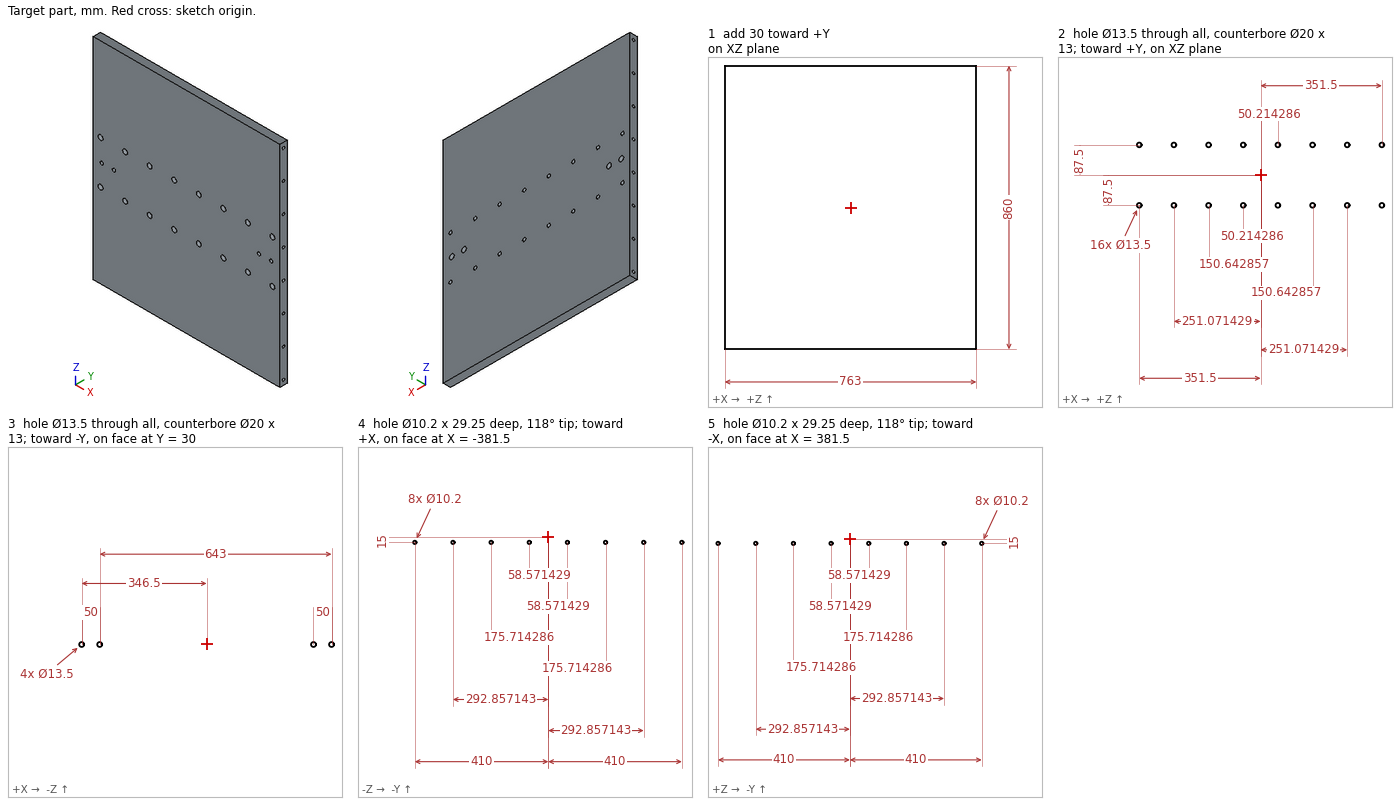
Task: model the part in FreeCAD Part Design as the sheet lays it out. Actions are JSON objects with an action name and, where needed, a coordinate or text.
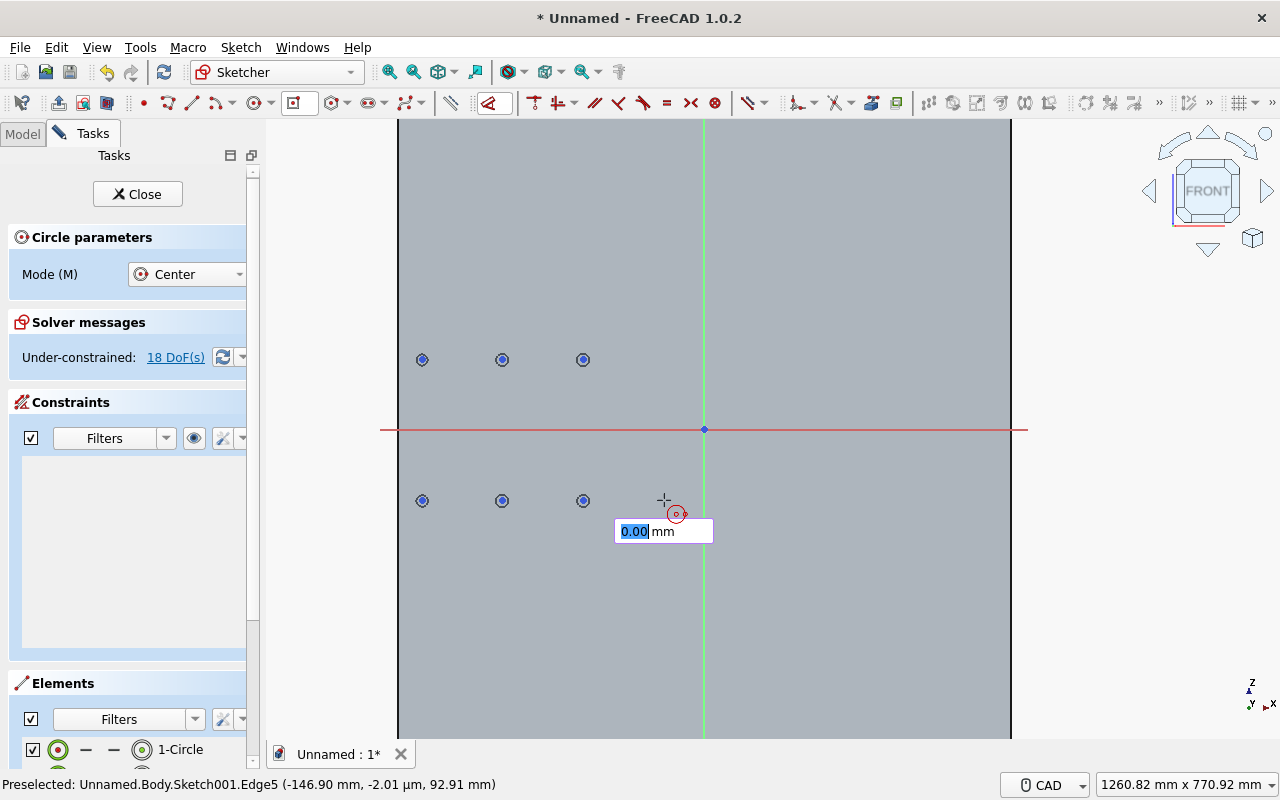
{"action": "scroll", "coordinate": [668, 496], "scroll_direction": "up", "scroll_amount": 6}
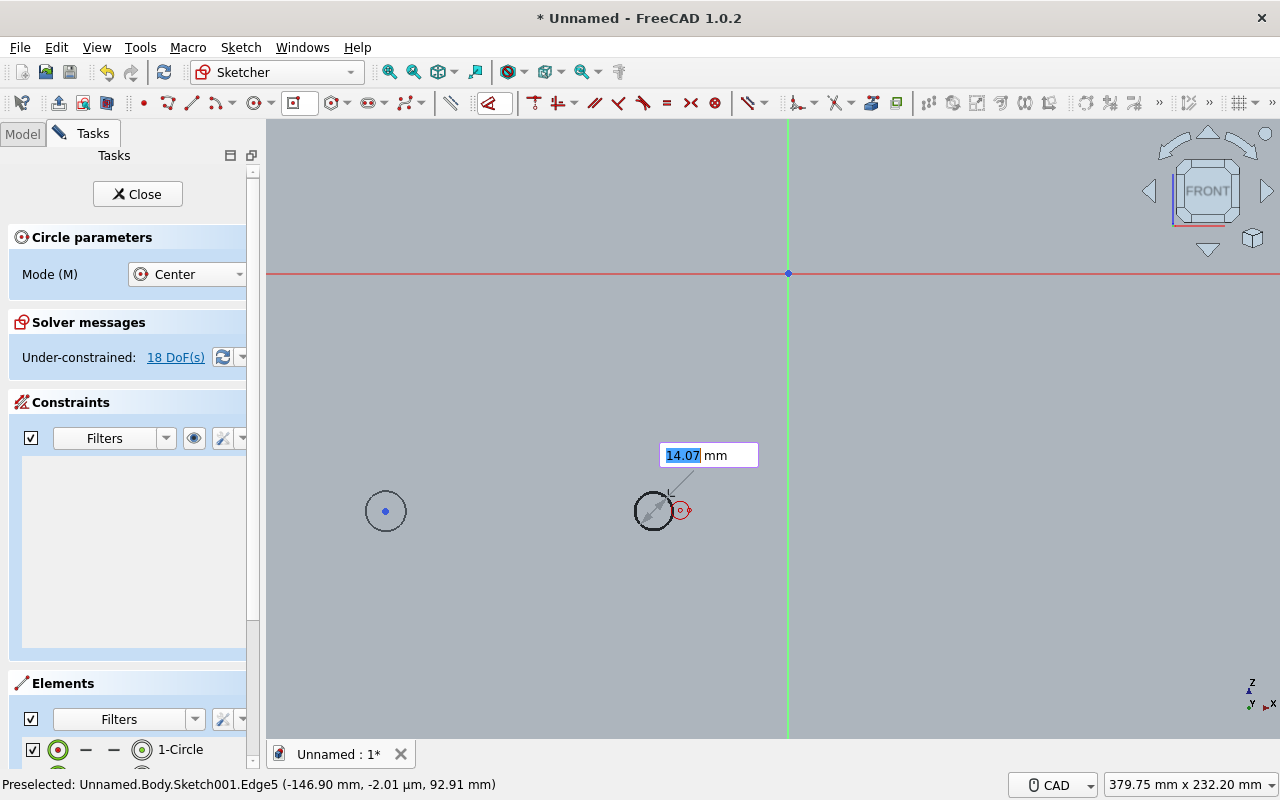
{"action": "left_click", "coordinate": [667, 495]}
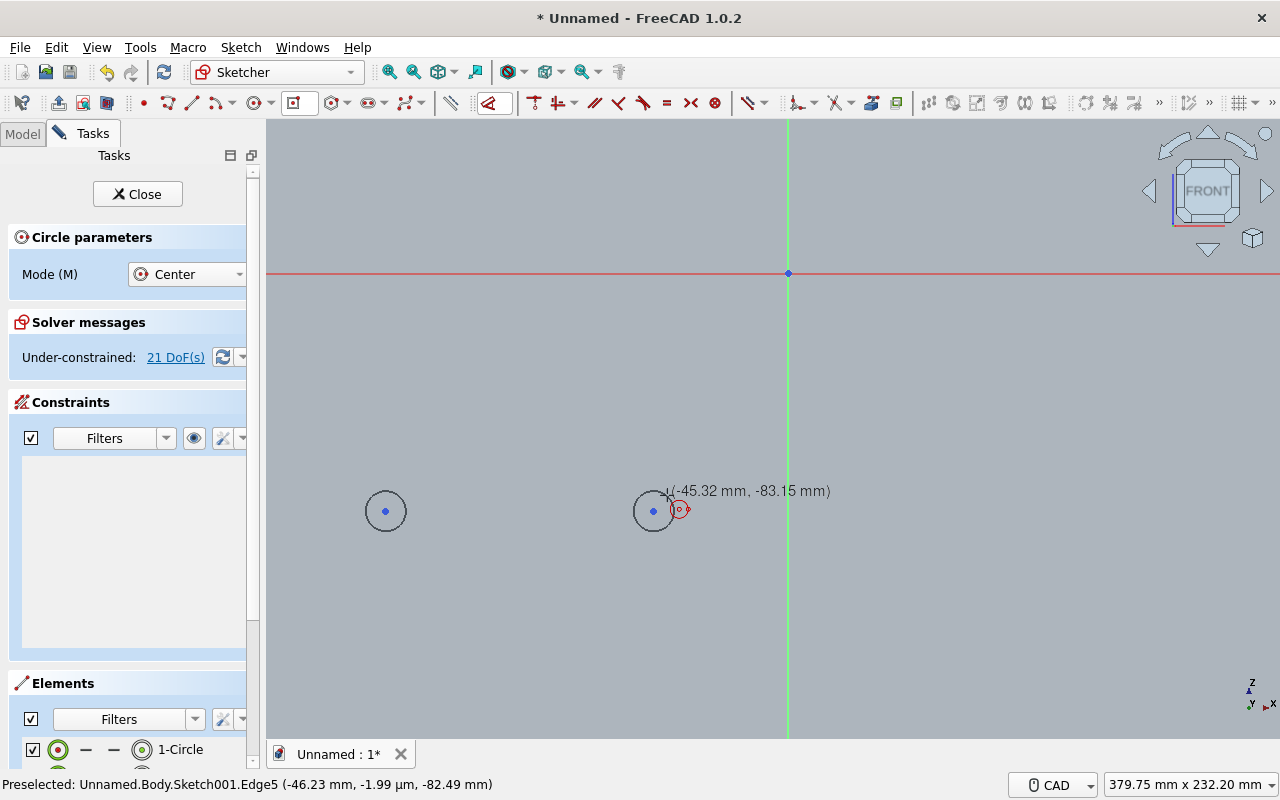
{"action": "scroll", "coordinate": [669, 496], "scroll_direction": "down", "scroll_amount": 6}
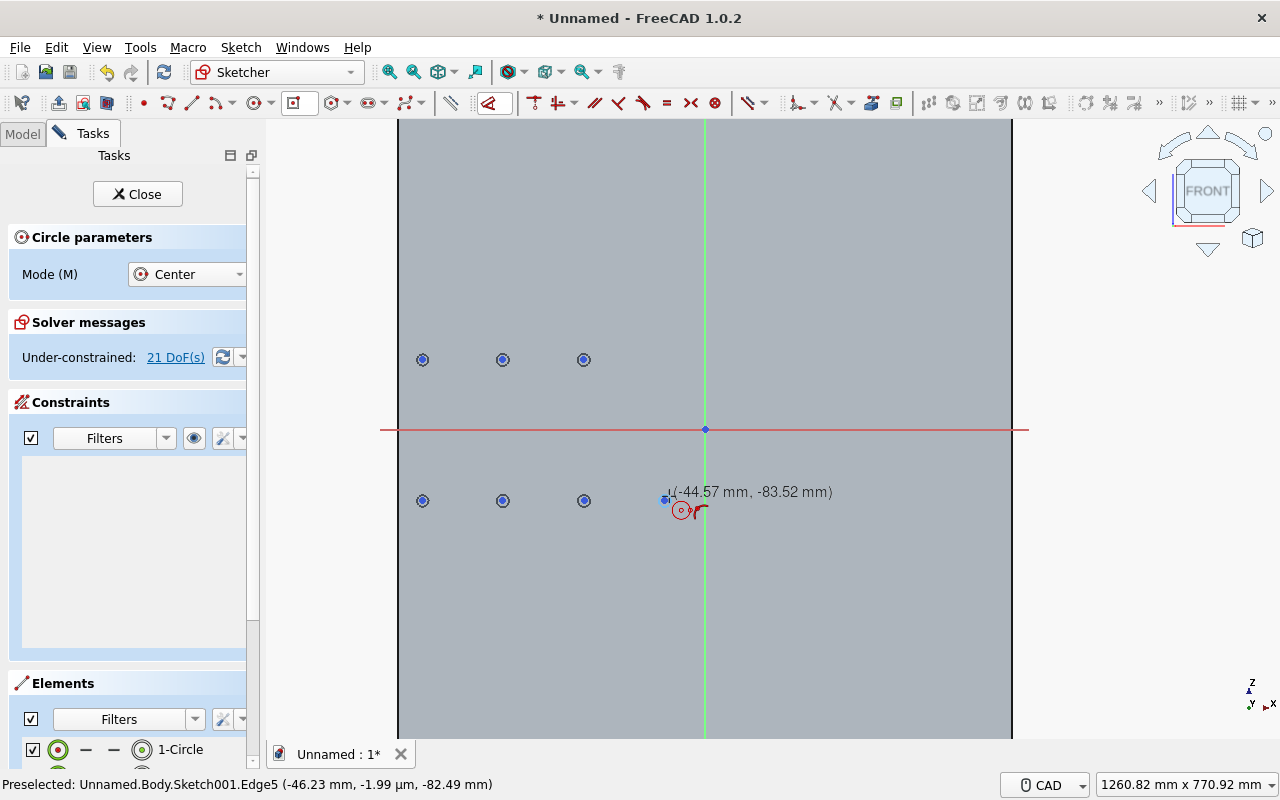
{"action": "scroll", "coordinate": [665, 359], "scroll_direction": "up", "scroll_amount": 8}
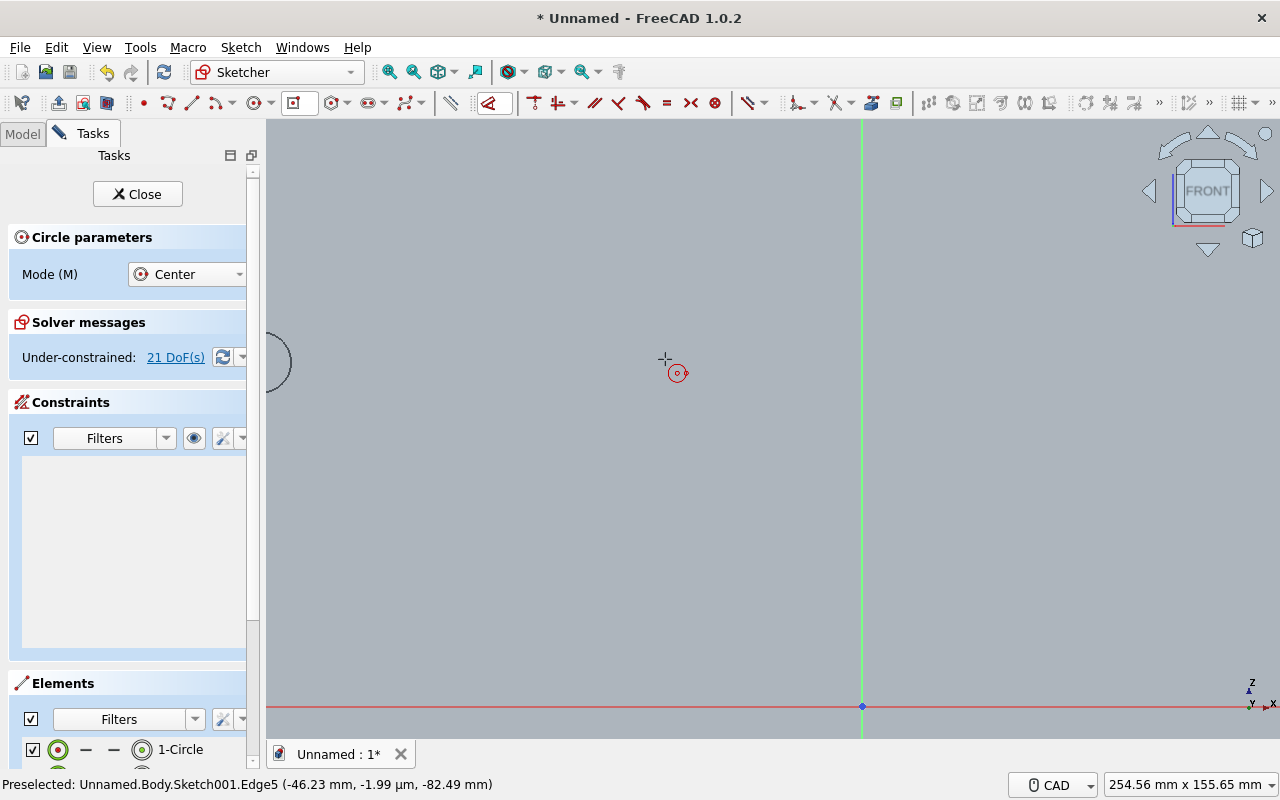
{"action": "scroll", "coordinate": [665, 359], "scroll_direction": "down", "scroll_amount": 8}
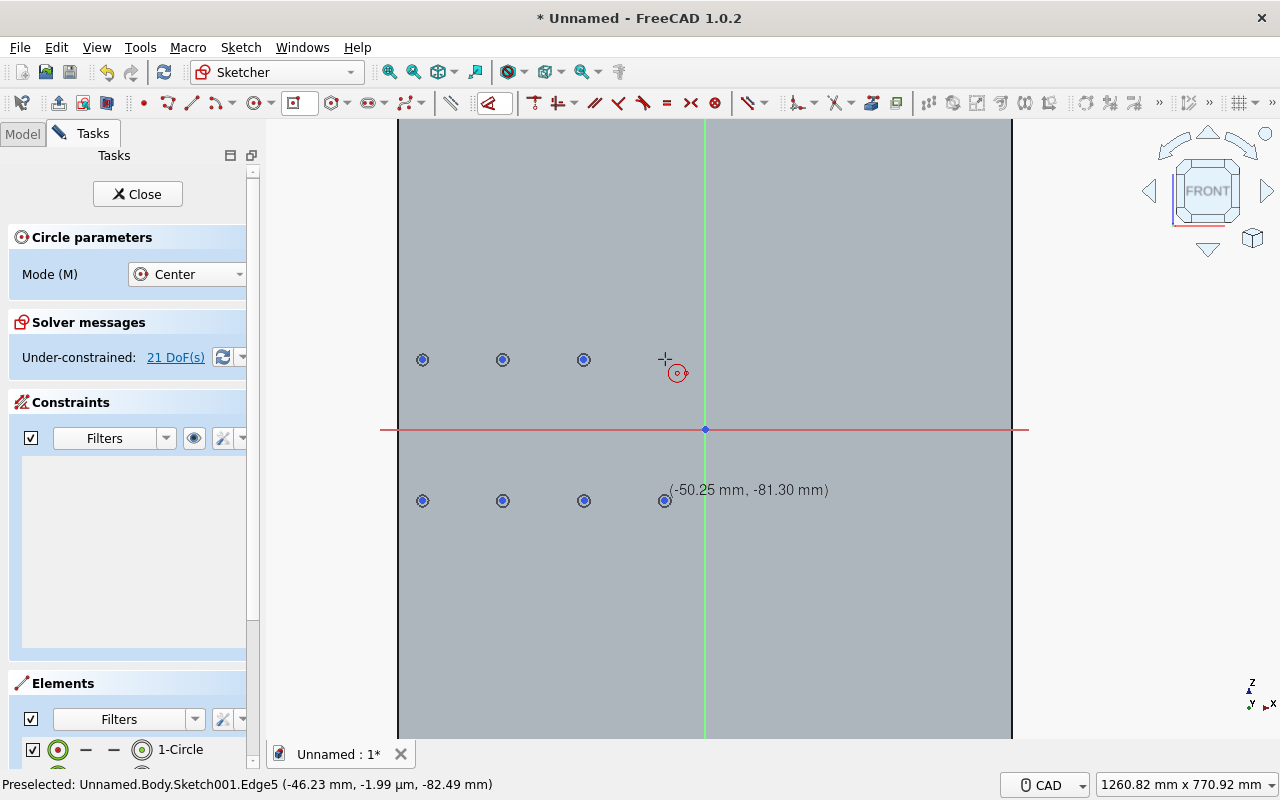
{"action": "left_click", "coordinate": [665, 359]}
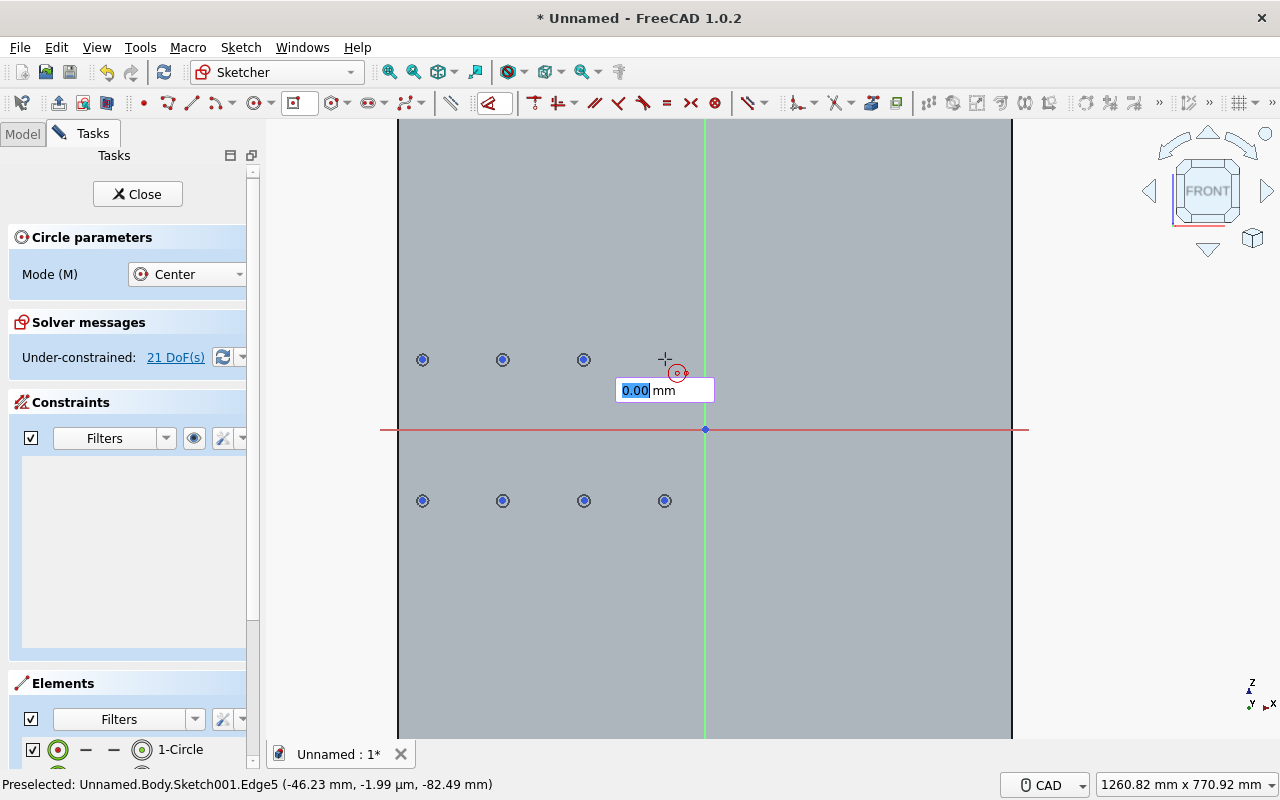
{"action": "scroll", "coordinate": [669, 355], "scroll_direction": "up", "scroll_amount": 6}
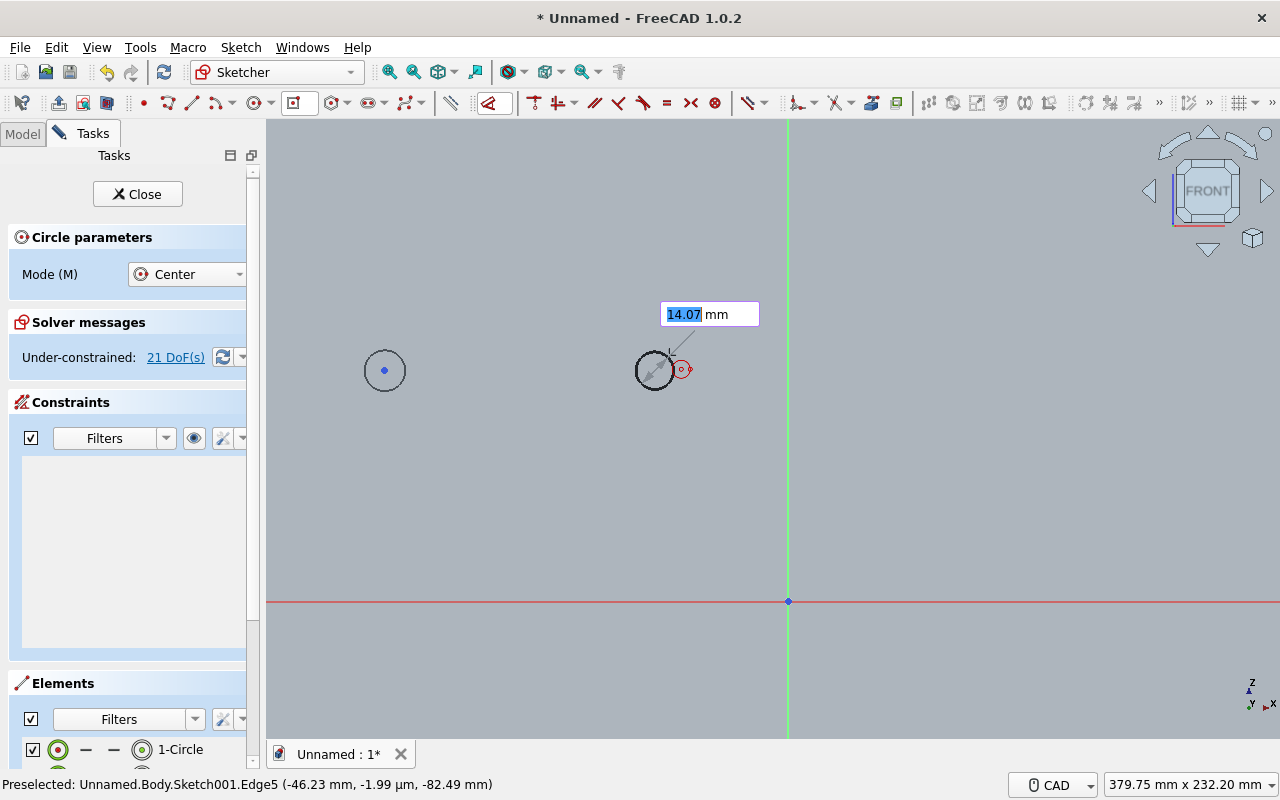
{"action": "left_click", "coordinate": [667, 355]}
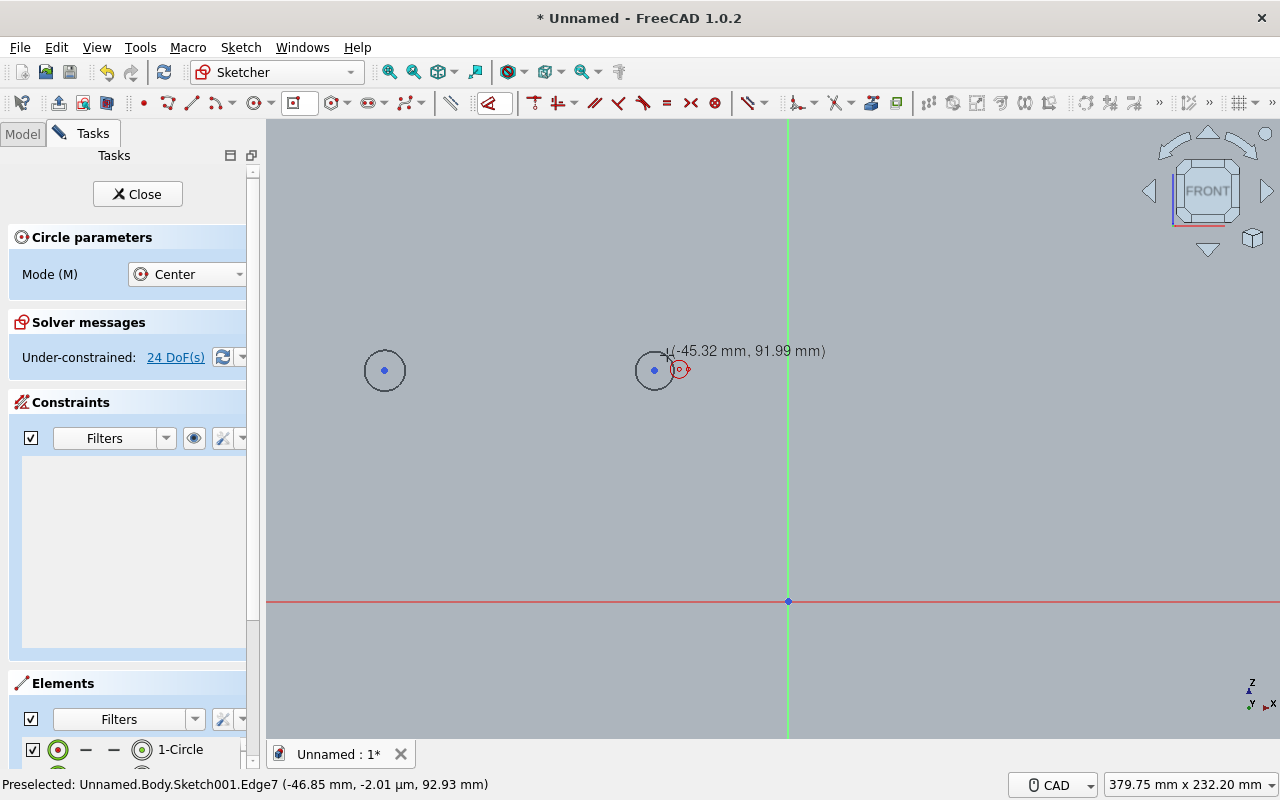
{"action": "scroll", "coordinate": [922, 368], "scroll_direction": "up", "scroll_amount": 2}